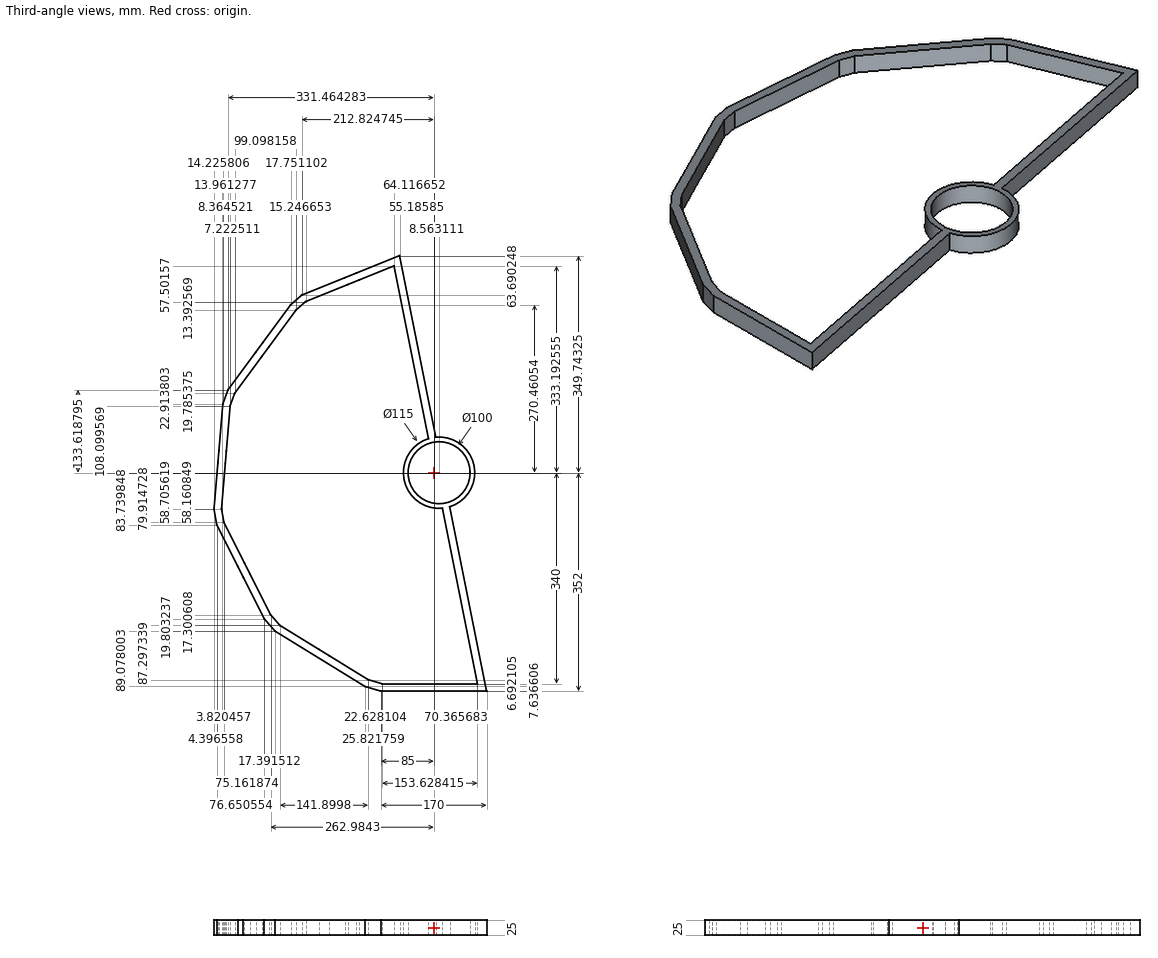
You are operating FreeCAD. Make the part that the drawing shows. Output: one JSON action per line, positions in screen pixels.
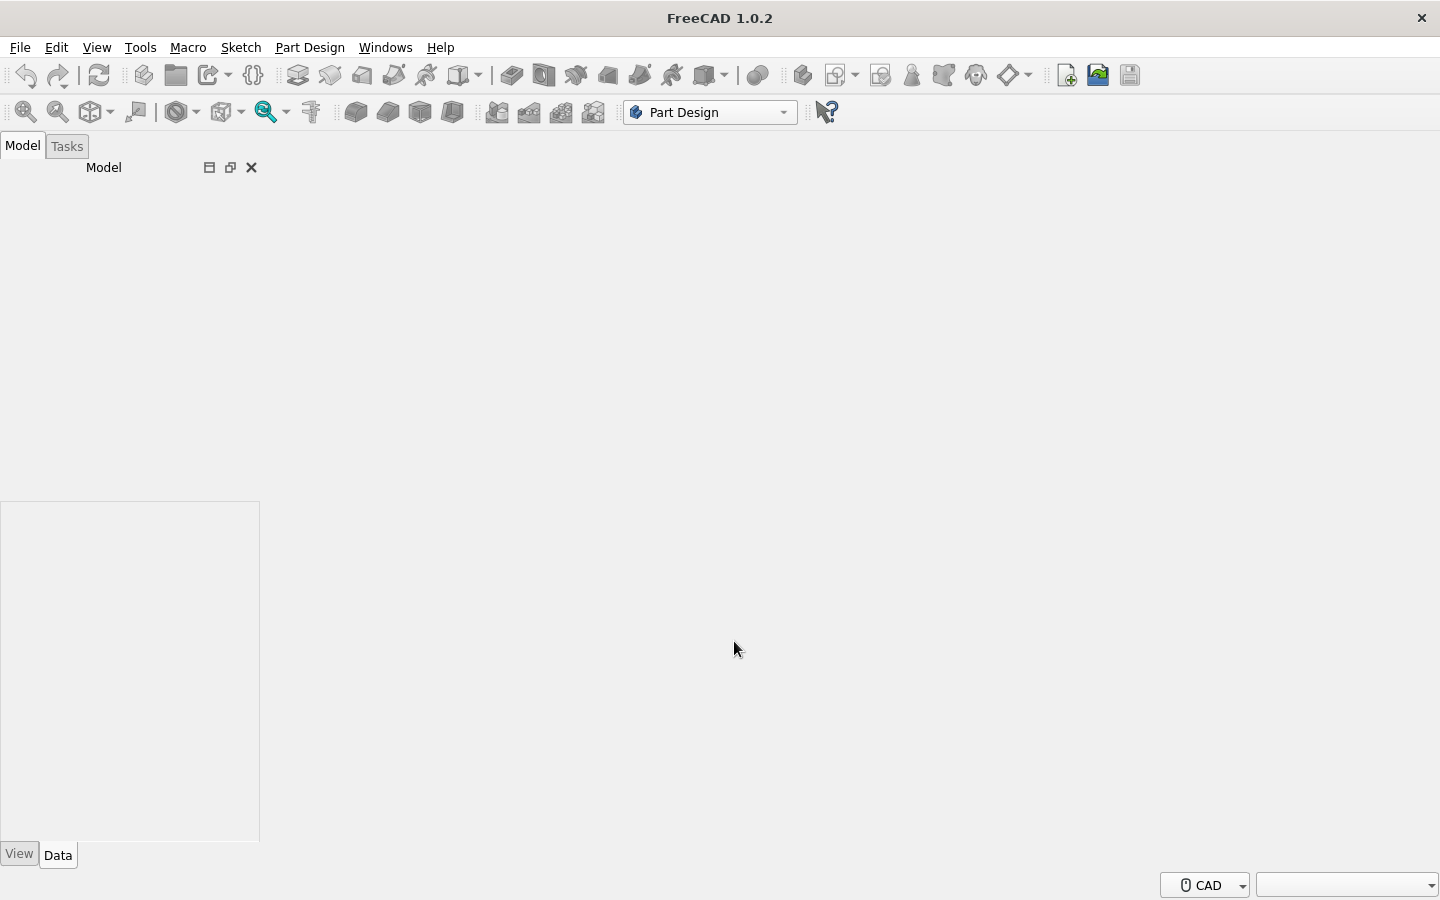
{"action": "left_click", "coordinate": [1066, 76]}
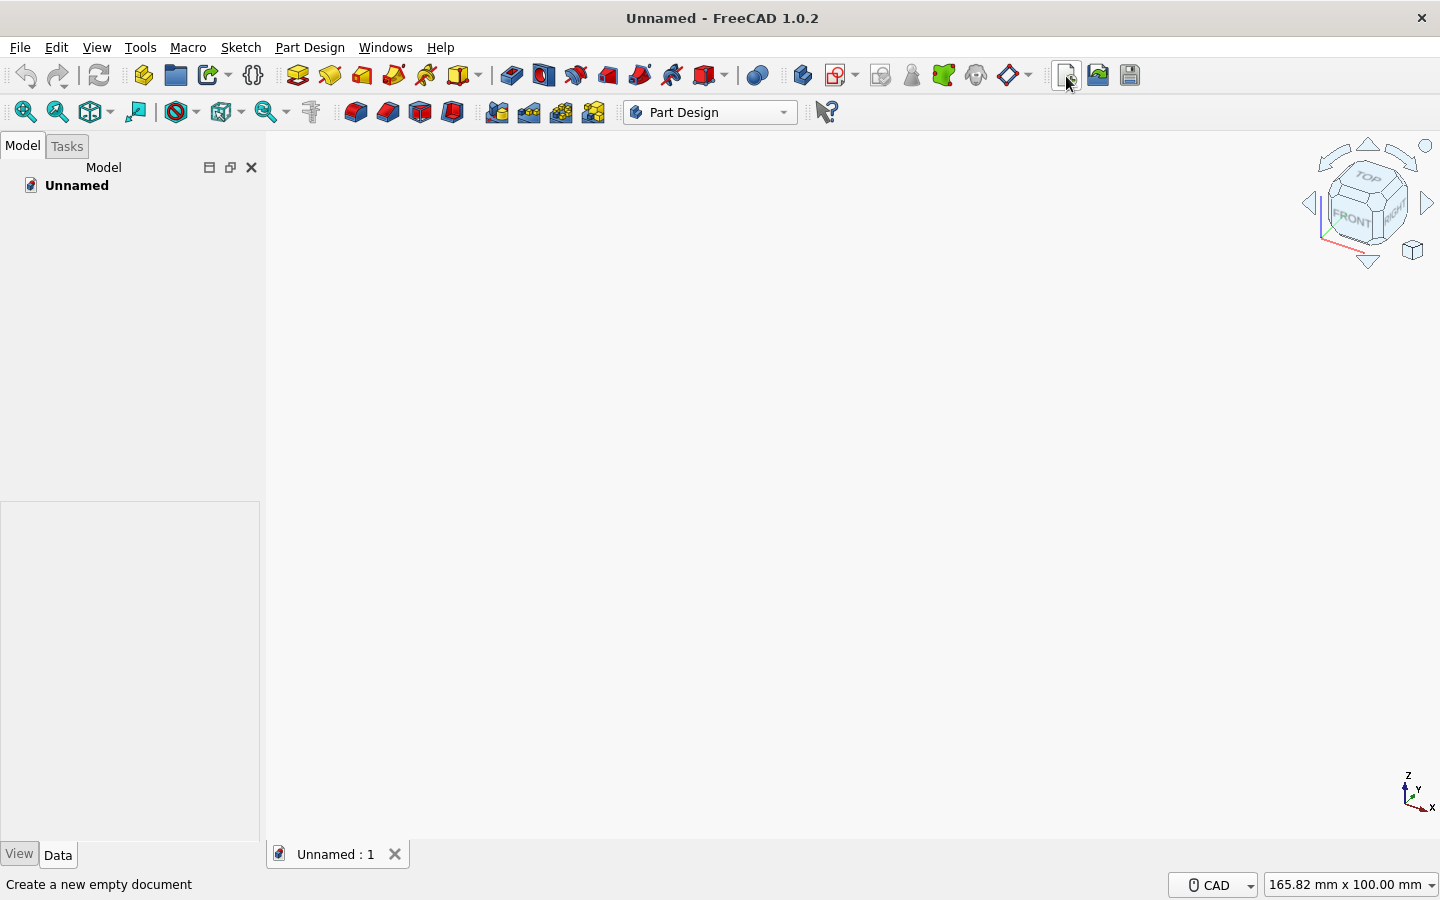
{"action": "left_click", "coordinate": [836, 76]}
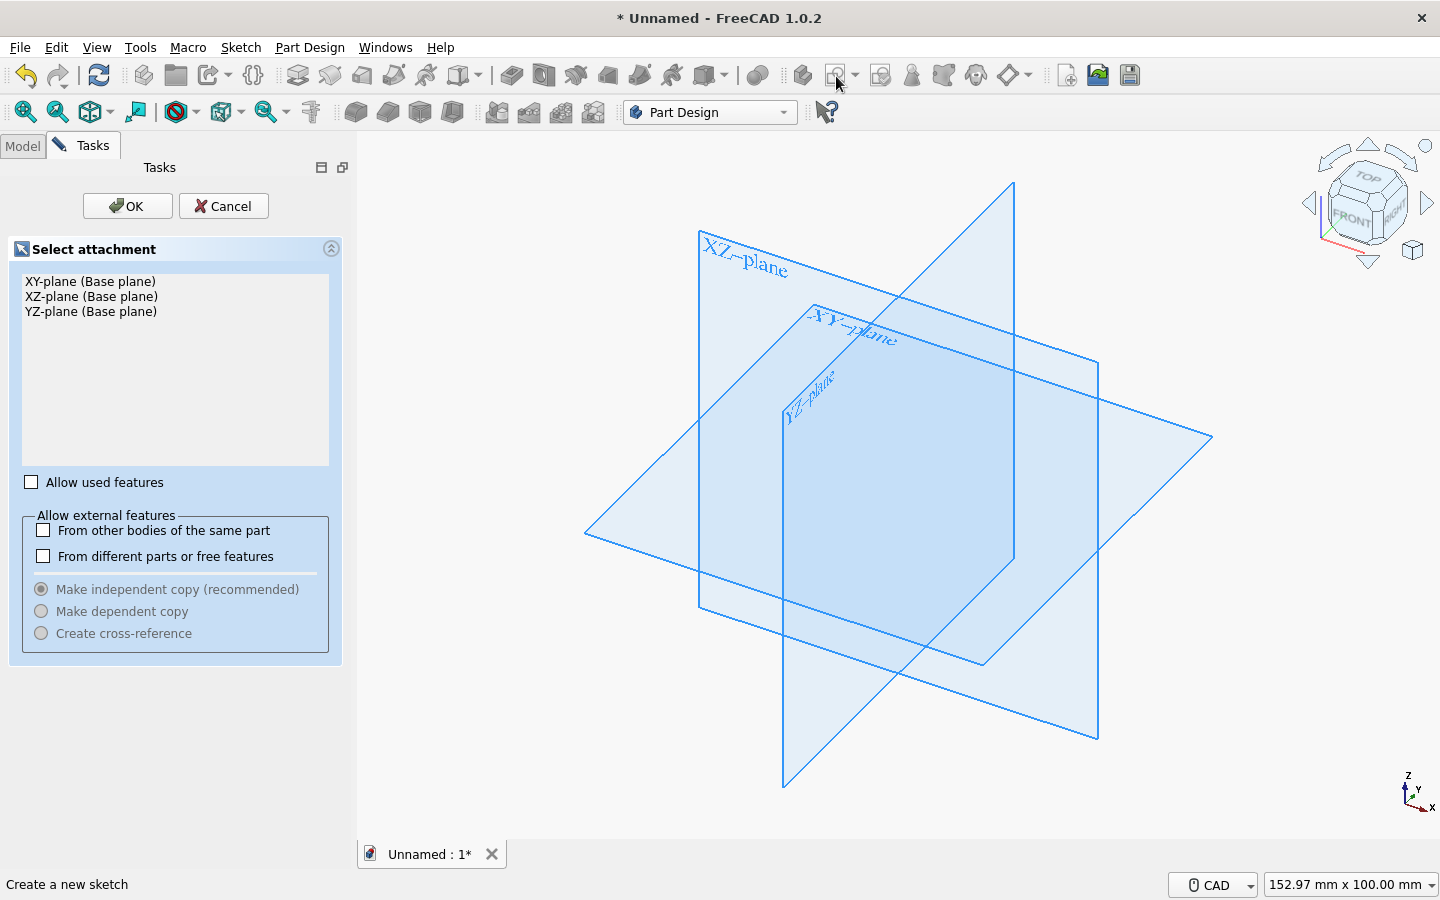
{"action": "left_click", "coordinate": [82, 282]}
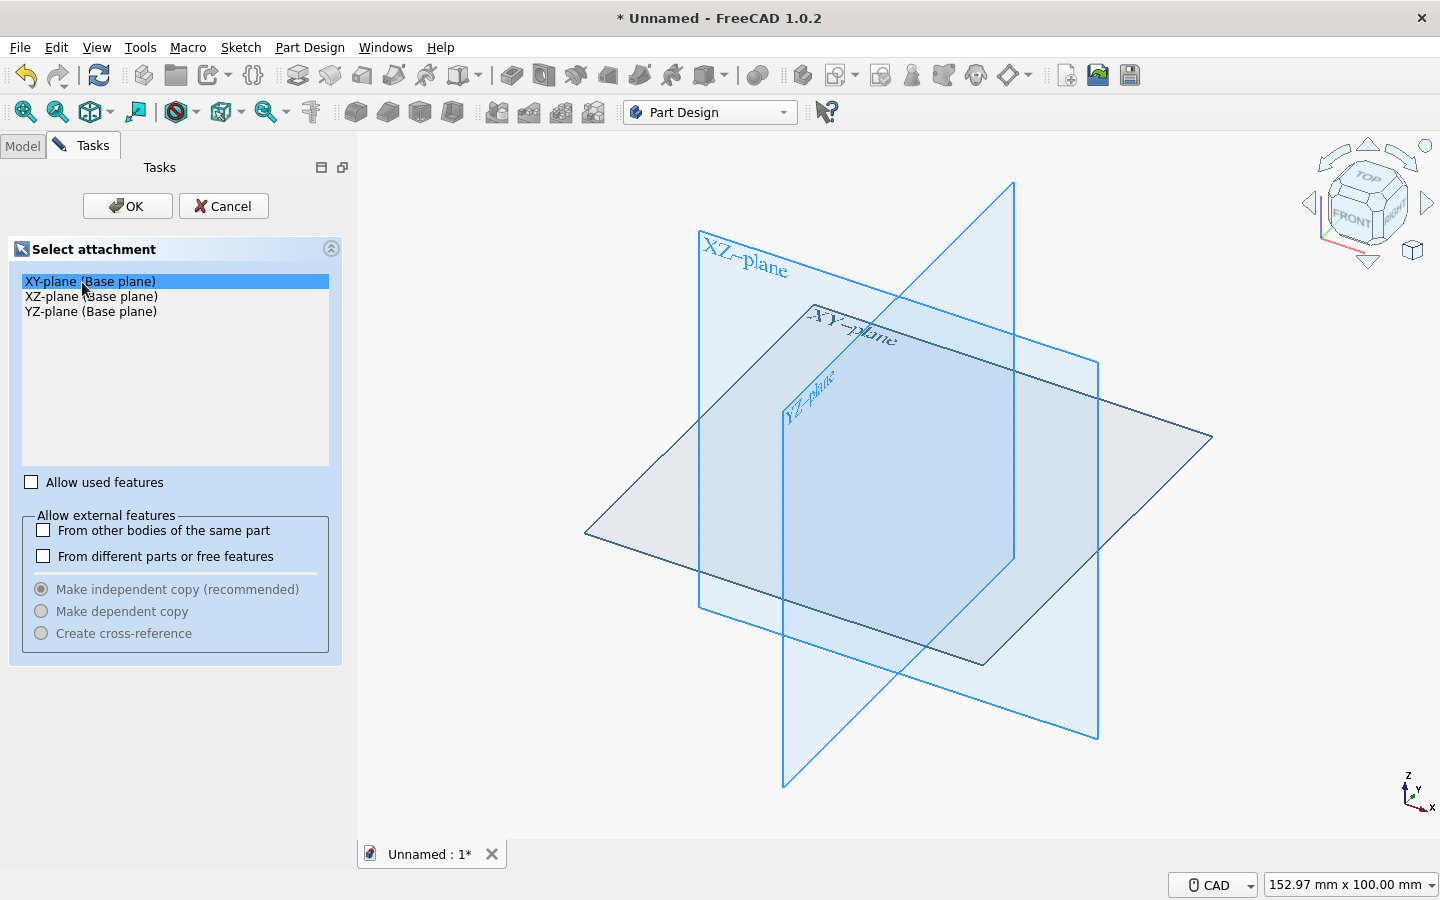
{"action": "left_click", "coordinate": [128, 206]}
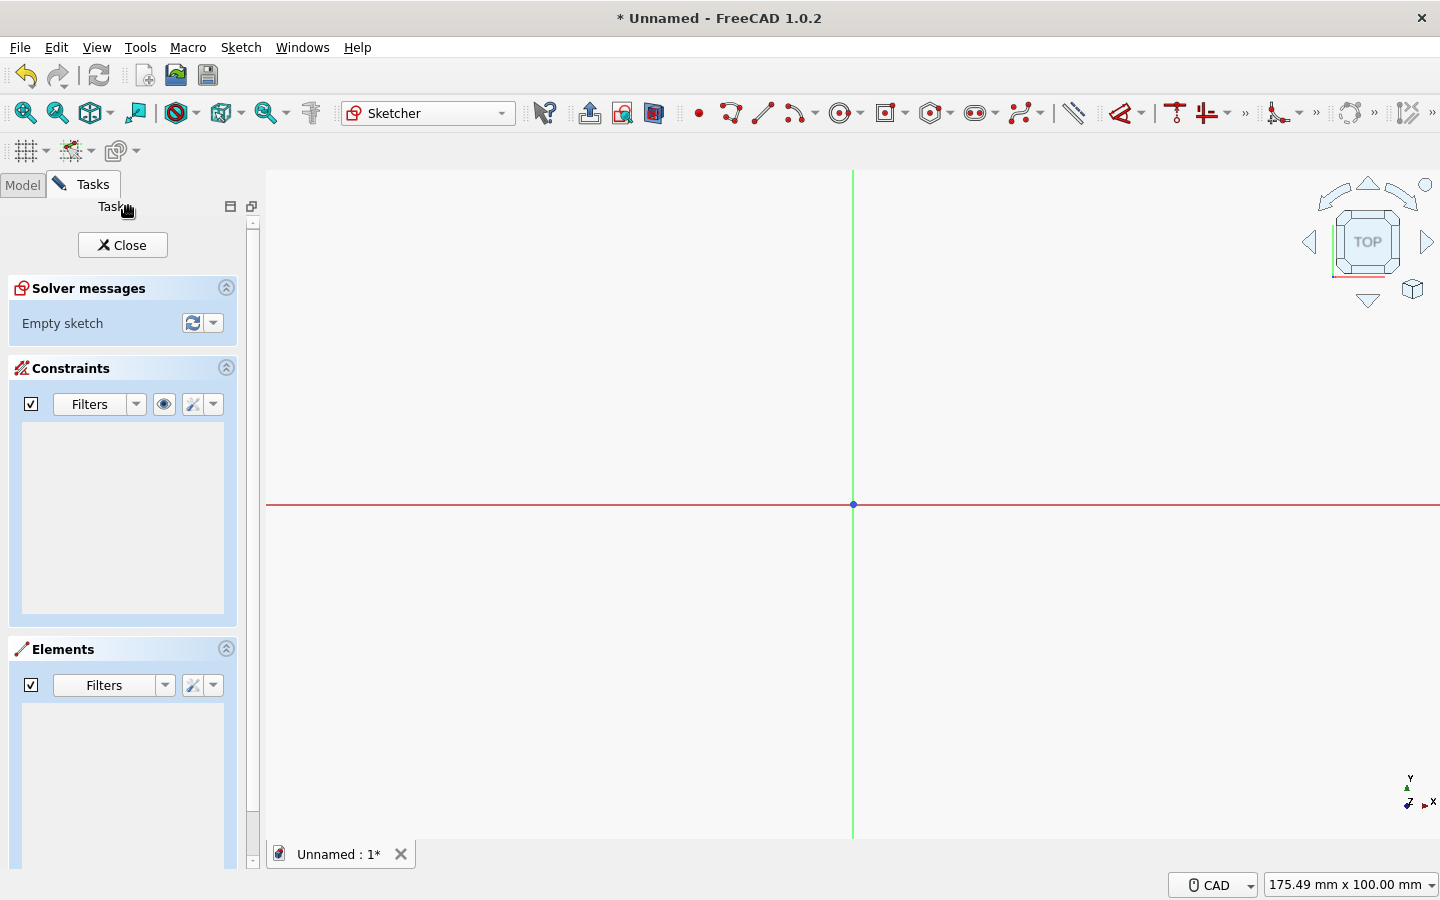
{"action": "scroll", "coordinate": [867, 504], "scroll_direction": "down", "scroll_amount": 12}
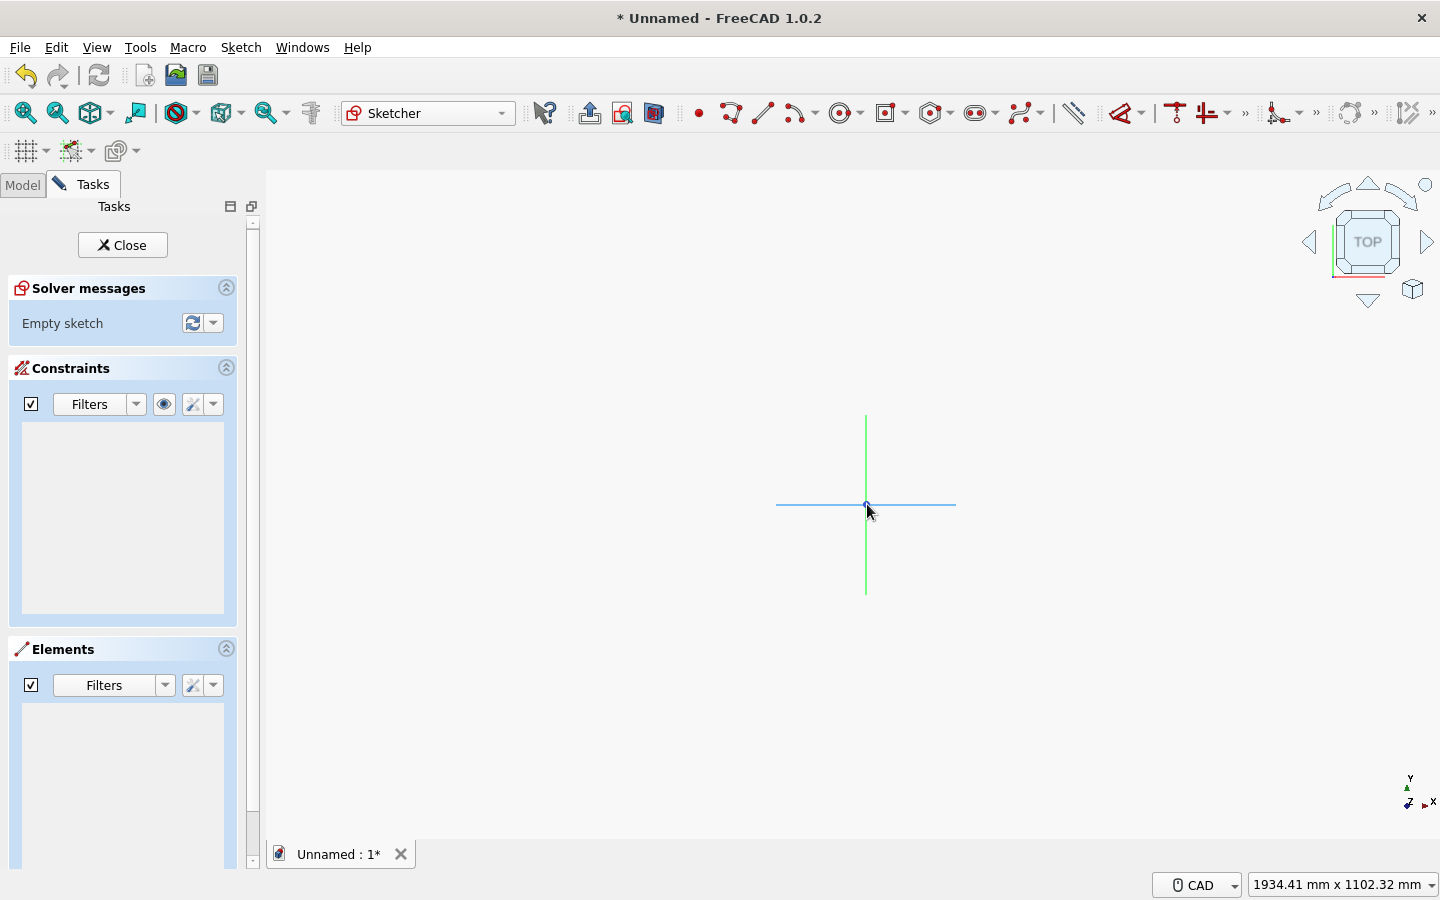
{"action": "left_click", "coordinate": [732, 114]}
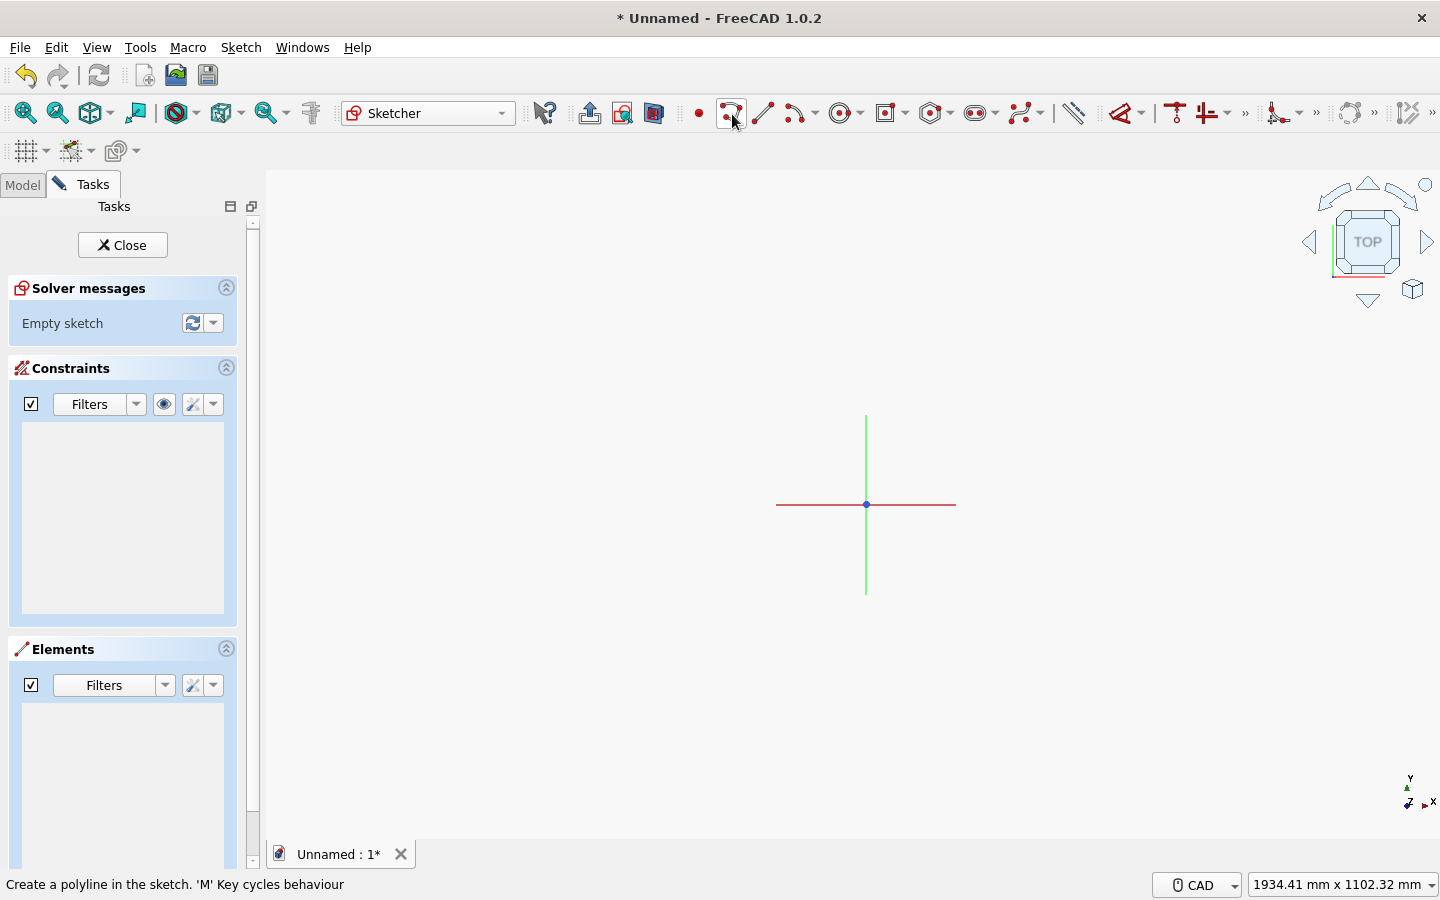
{"action": "left_click", "coordinate": [833, 292]}
{"action": "left_click", "coordinate": [737, 331]}
{"action": "left_click", "coordinate": [726, 340]}
{"action": "left_click", "coordinate": [665, 423]}
{"action": "left_click", "coordinate": [660, 437]}
{"action": "left_click", "coordinate": [651, 540]}
{"action": "left_click", "coordinate": [654, 555]}
{"action": "left_click", "coordinate": [701, 647]}
{"action": "left_click", "coordinate": [711, 659]}
{"action": "left_click", "coordinate": [799, 713]}
{"action": "left_click", "coordinate": [815, 718]}
{"action": "left_click", "coordinate": [918, 718]}
{"action": "left_click", "coordinate": [833, 293]}